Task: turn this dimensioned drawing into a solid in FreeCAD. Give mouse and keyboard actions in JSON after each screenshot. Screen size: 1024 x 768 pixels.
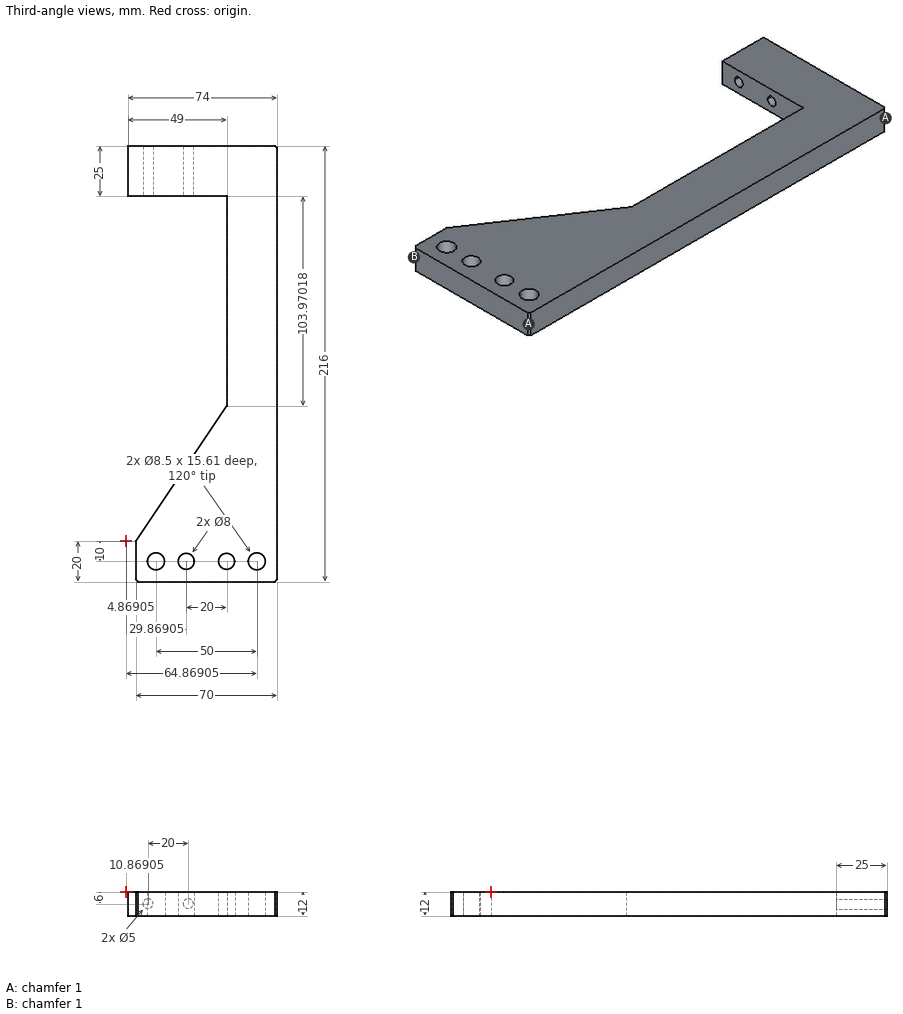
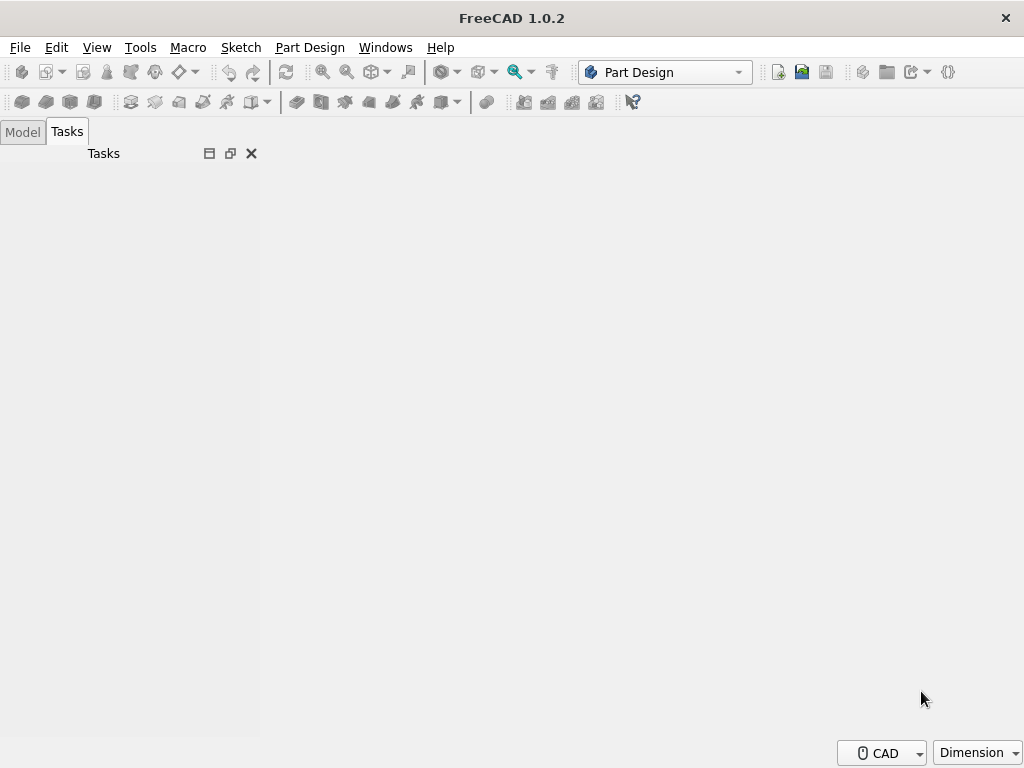
{"action": "key", "text": "ctrl+n"}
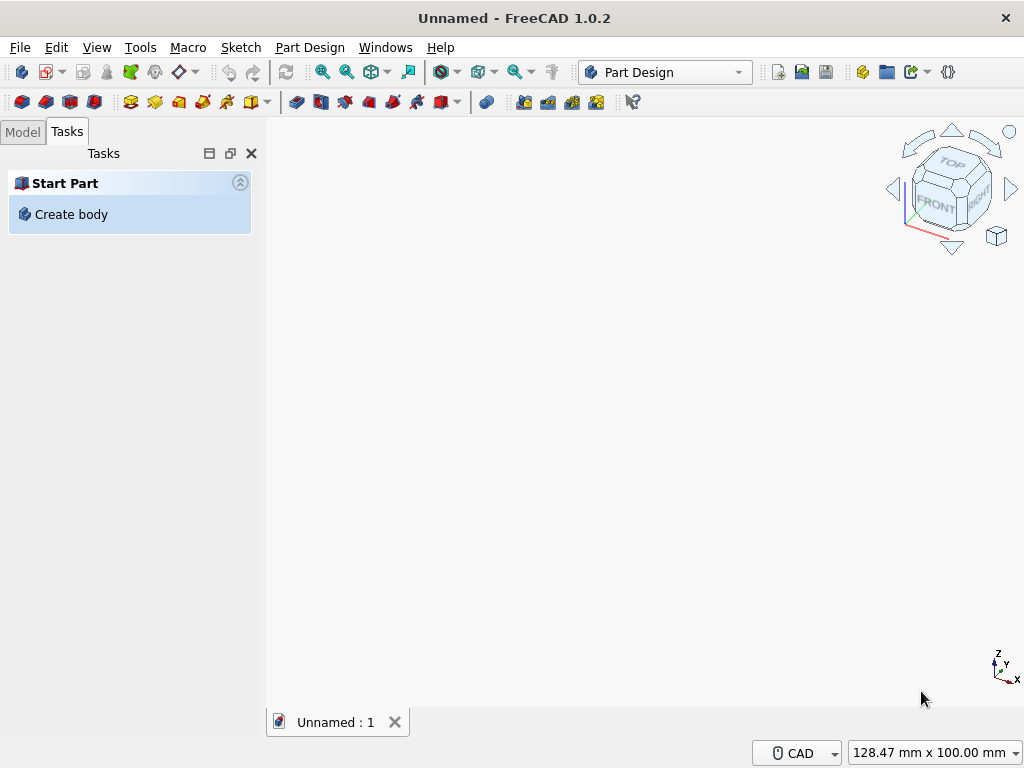
{"action": "left_click", "coordinate": [46, 72]}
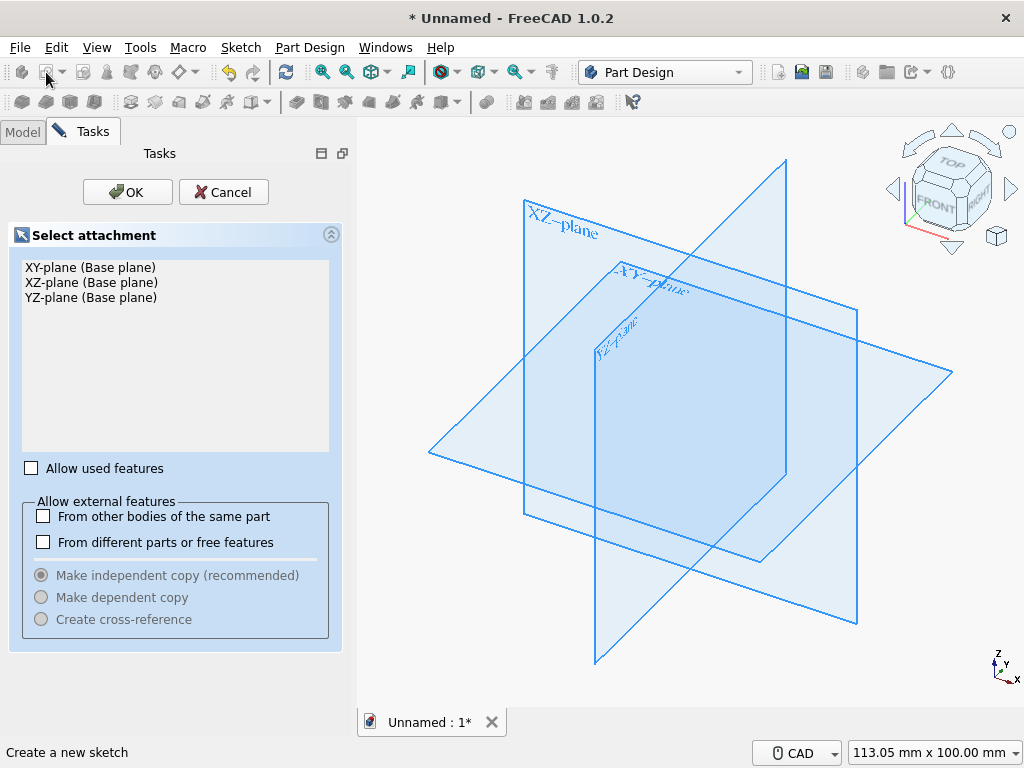
{"action": "left_click", "coordinate": [82, 268]}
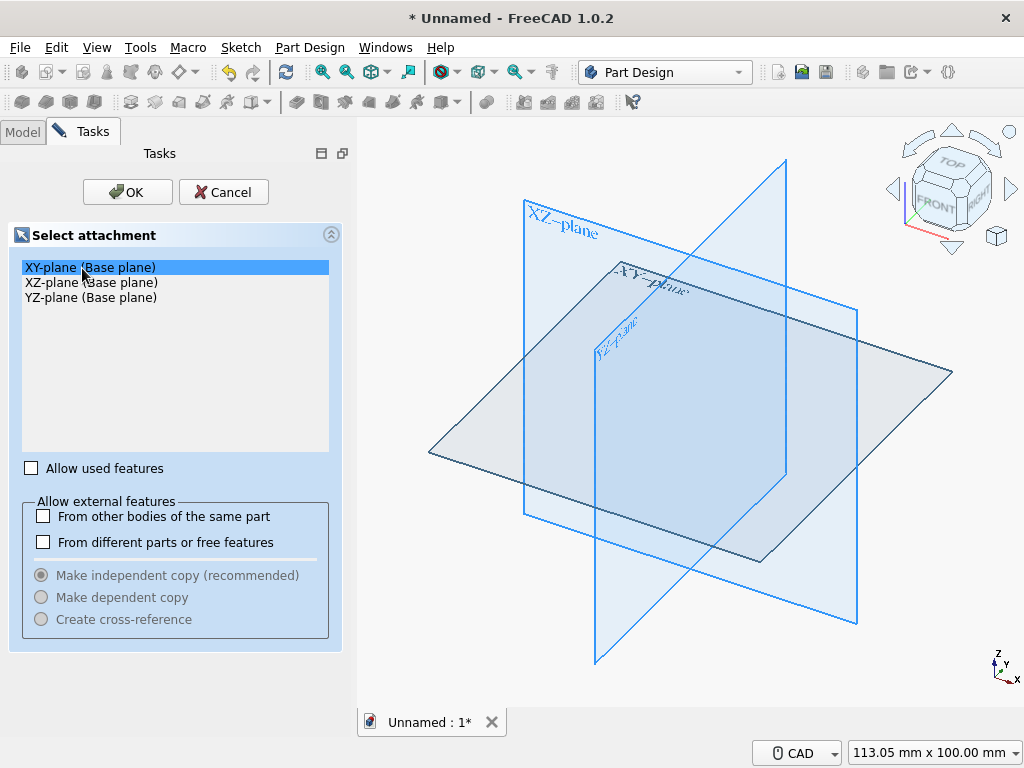
{"action": "left_click", "coordinate": [128, 192]}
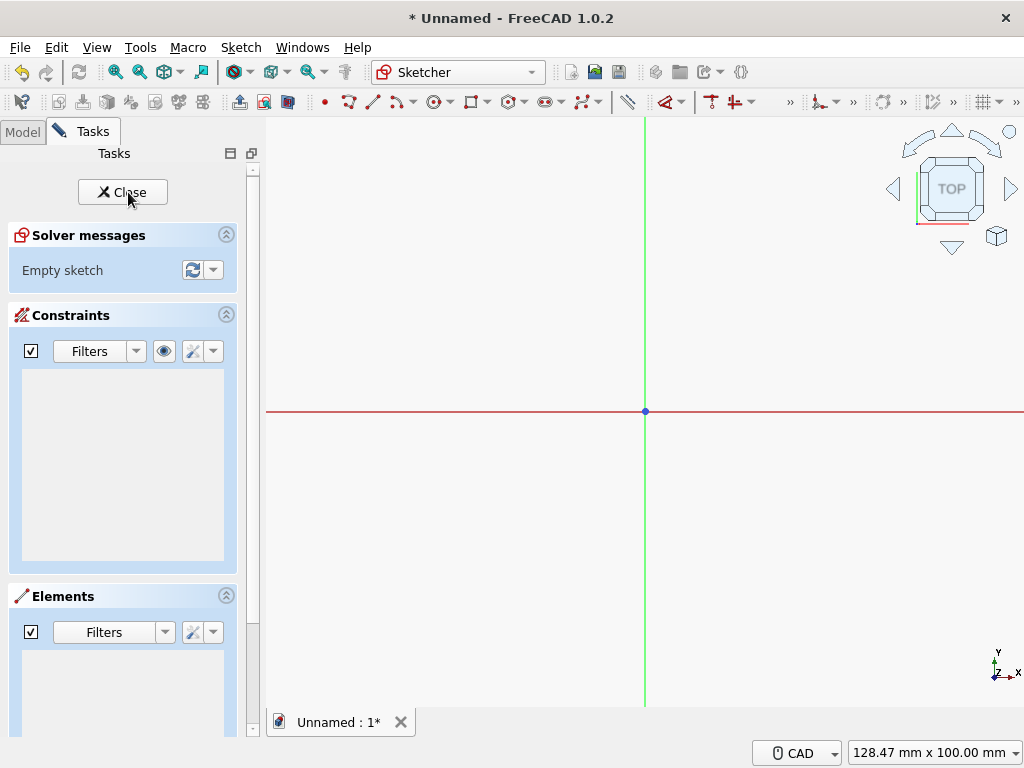
{"action": "scroll", "coordinate": [452, 636], "scroll_direction": "down", "scroll_amount": 6}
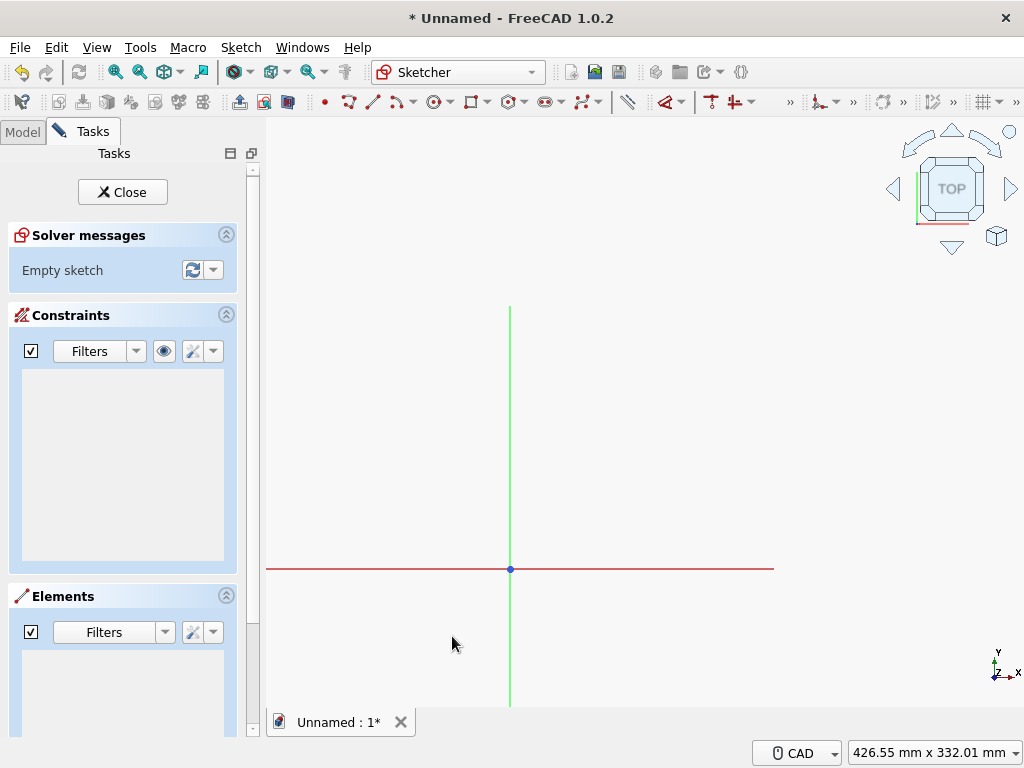
{"action": "key", "text": "g m"}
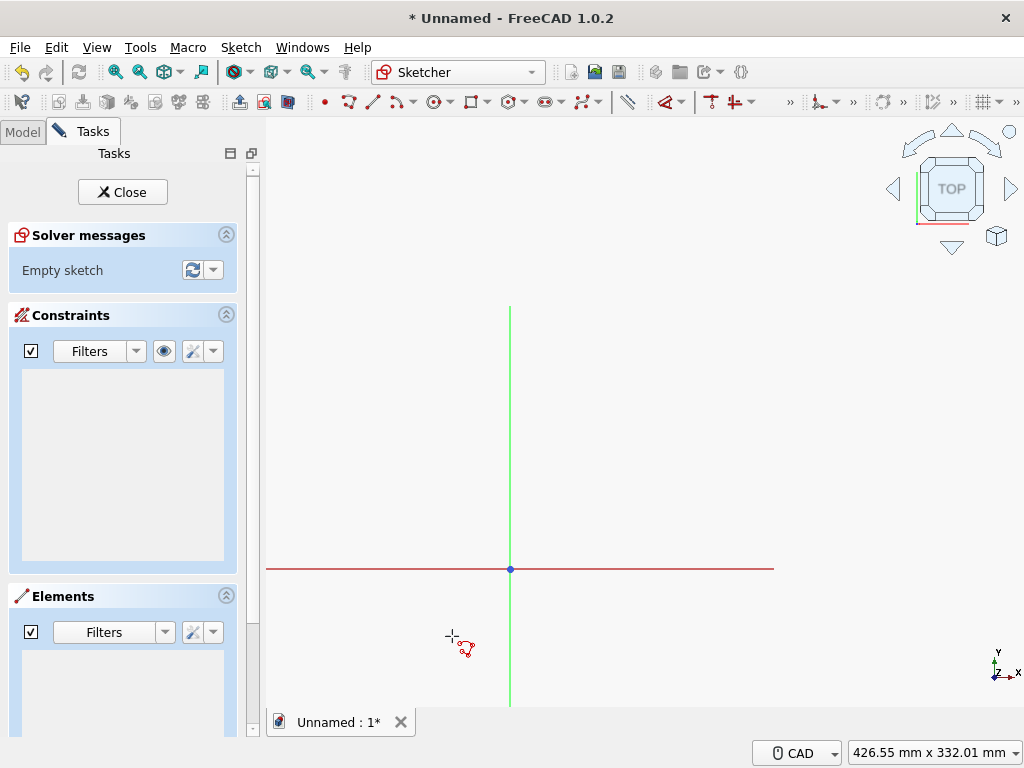
{"action": "scroll", "coordinate": [519, 569], "scroll_direction": "up", "scroll_amount": 4}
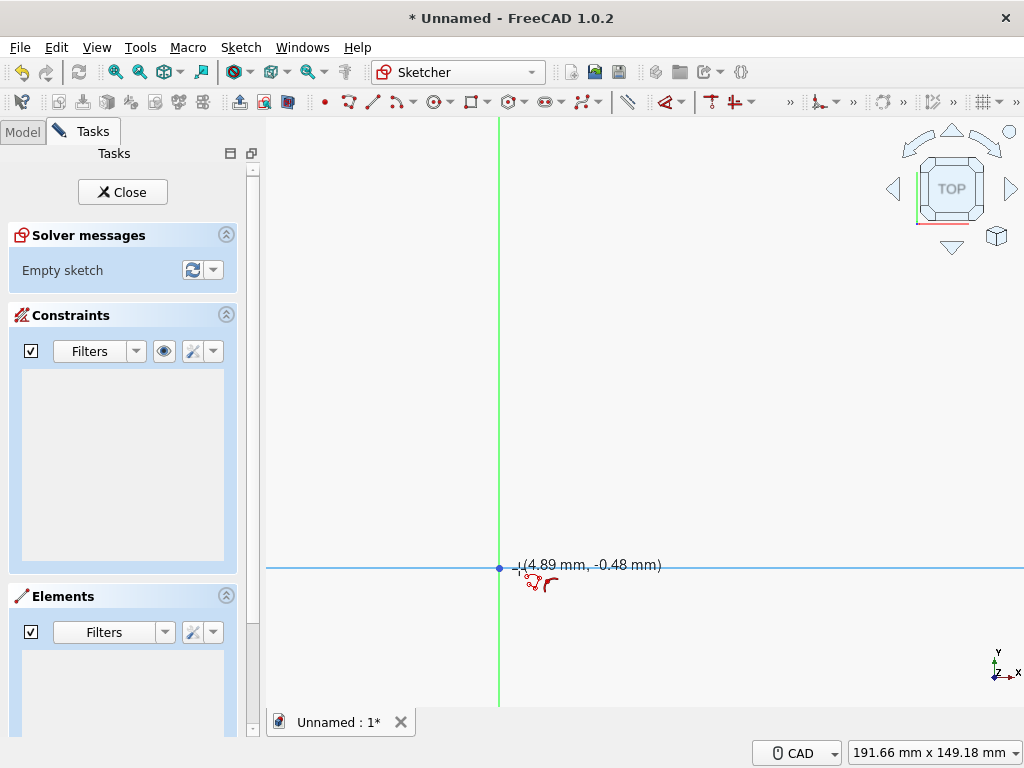
{"action": "left_click", "coordinate": [518, 568]}
{"action": "left_click", "coordinate": [518, 647]}
{"action": "left_click", "coordinate": [795, 647]}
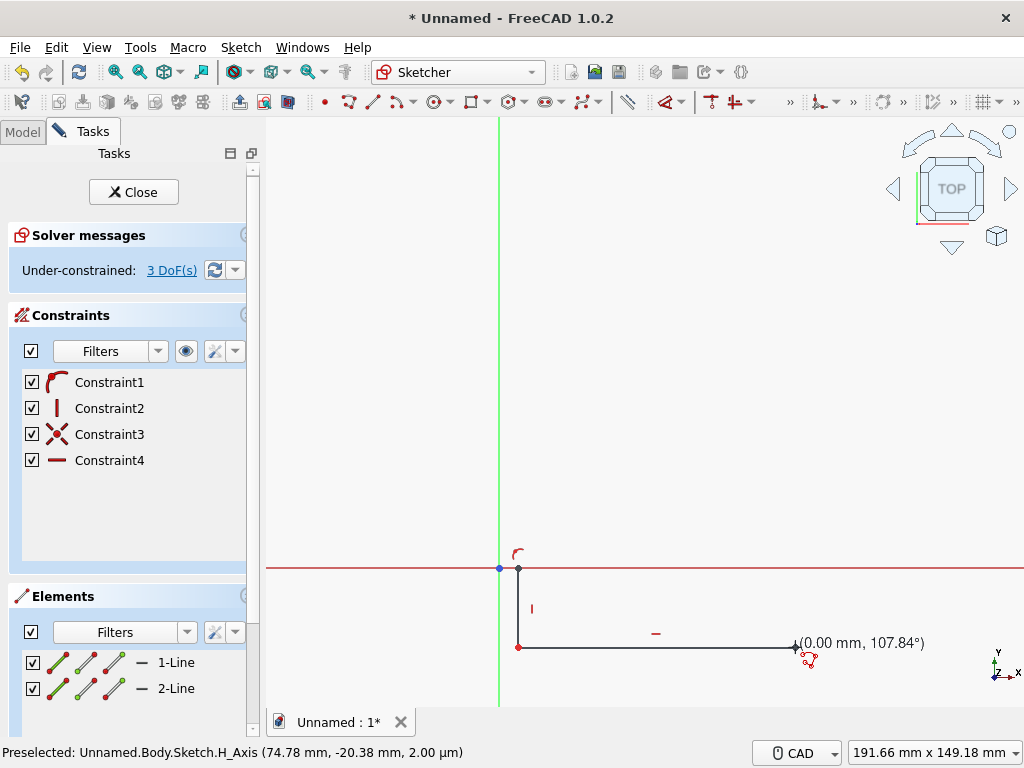
{"action": "scroll", "coordinate": [519, 568], "scroll_direction": "down", "scroll_amount": 4}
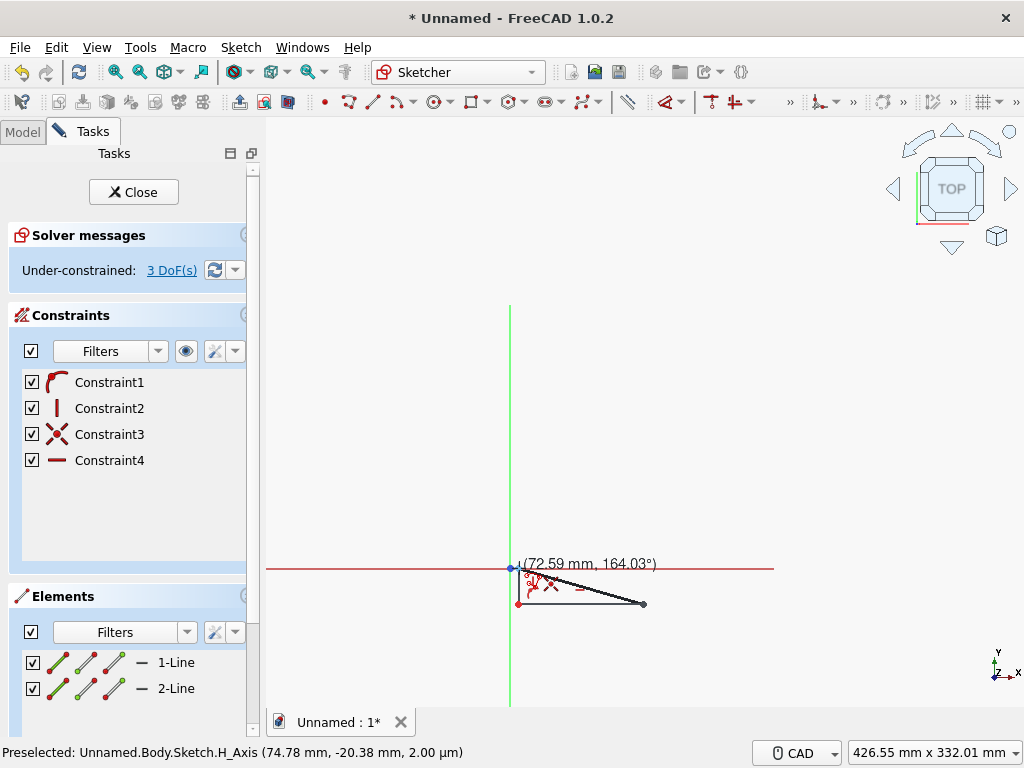
{"action": "left_click", "coordinate": [643, 220]}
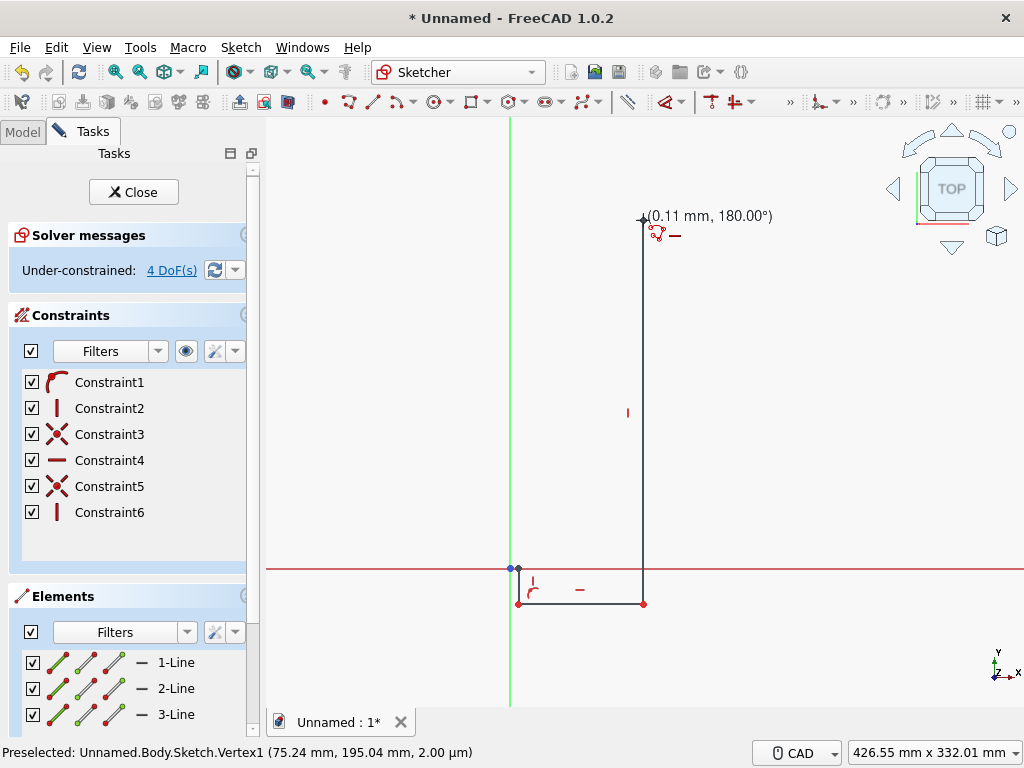
{"action": "scroll", "coordinate": [512, 220], "scroll_direction": "up", "scroll_amount": 12}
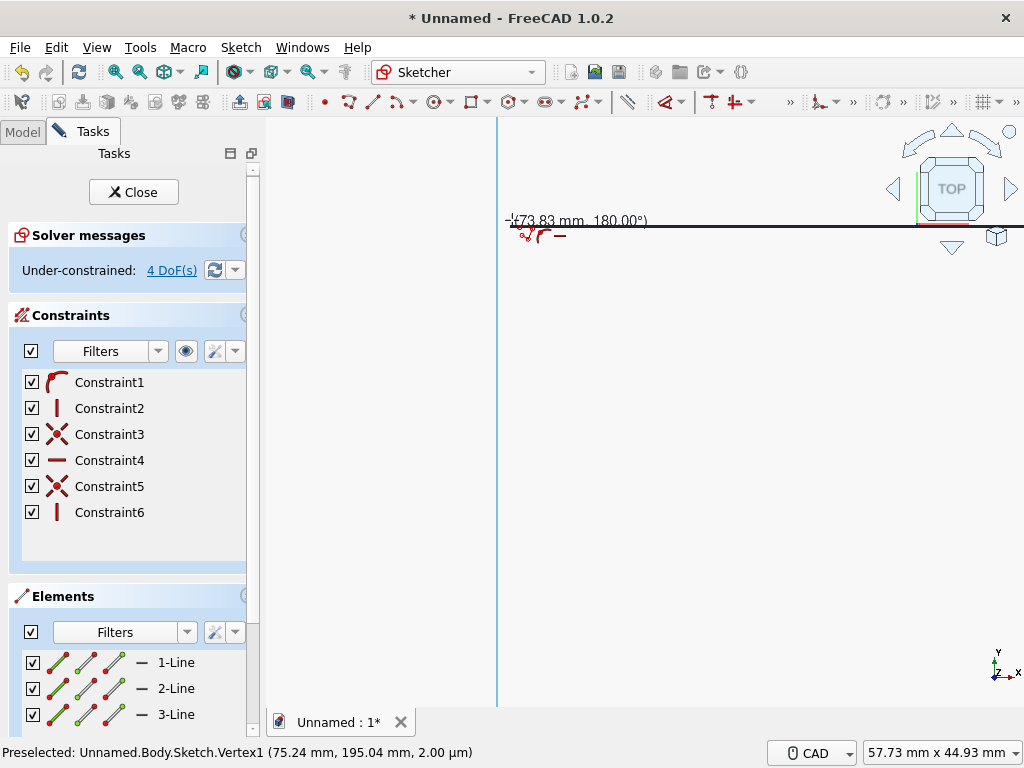
{"action": "left_click", "coordinate": [507, 218]}